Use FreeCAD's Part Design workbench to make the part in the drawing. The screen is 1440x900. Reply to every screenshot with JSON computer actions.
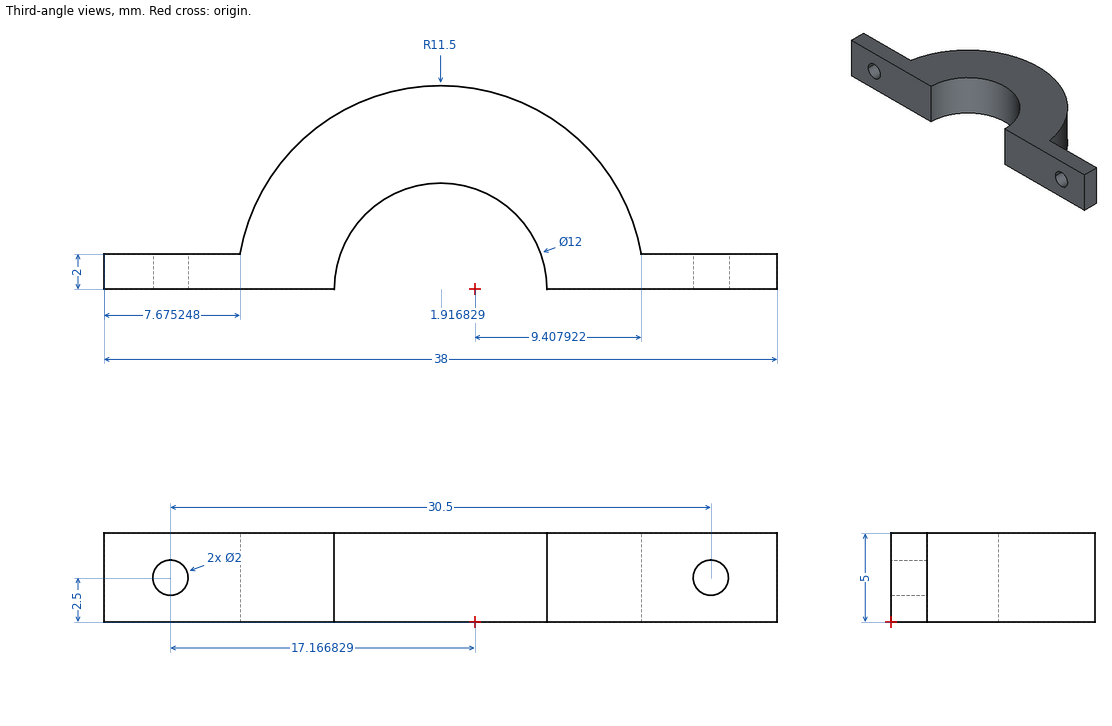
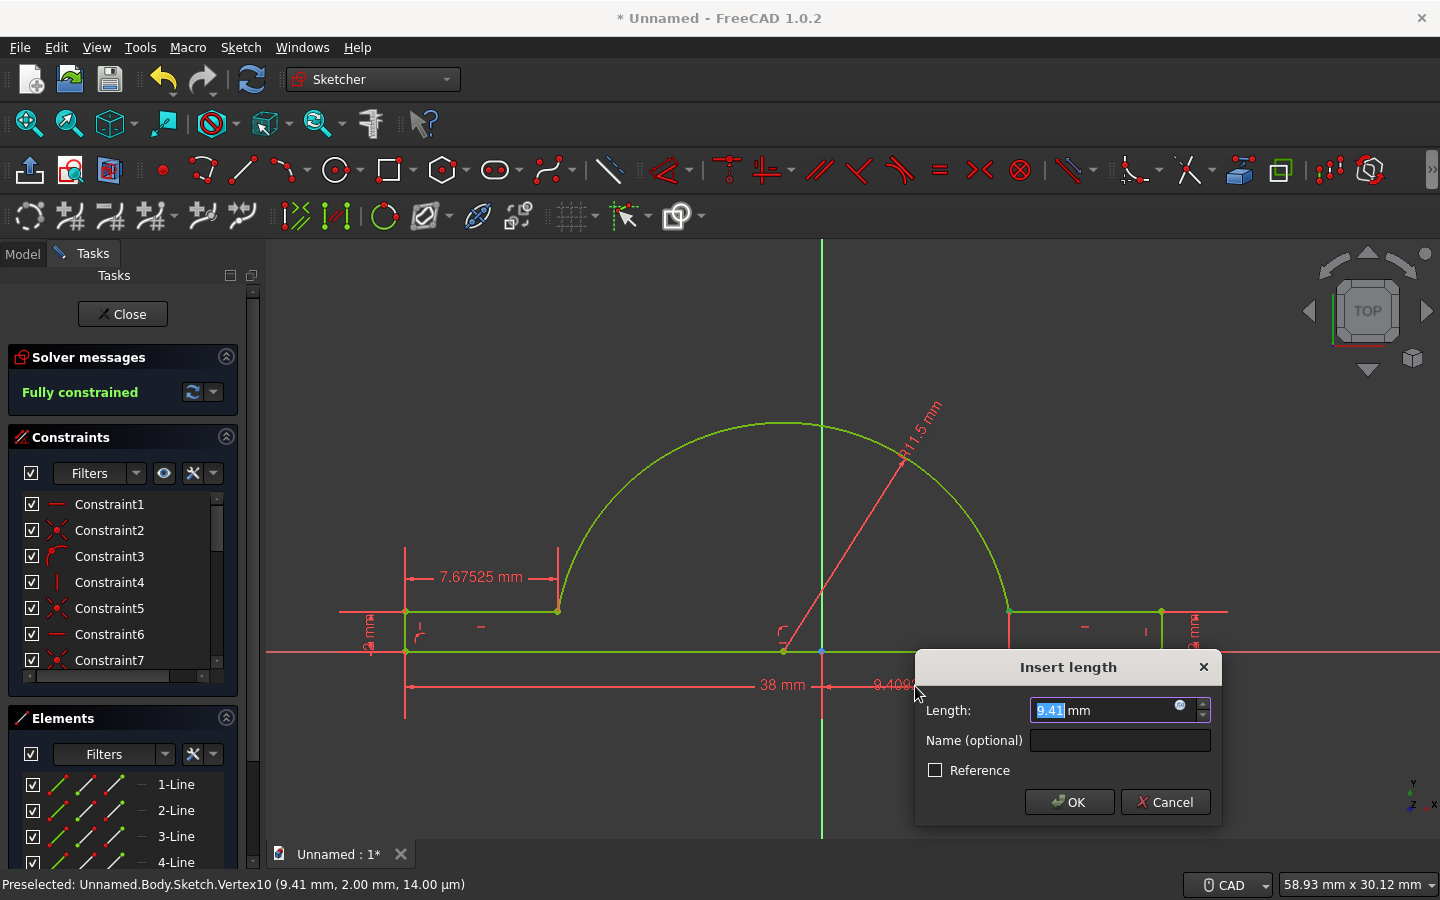
{"action": "type", "text": "9.407922"}
{"action": "key", "text": "Return"}
{"action": "key", "text": "Escape"}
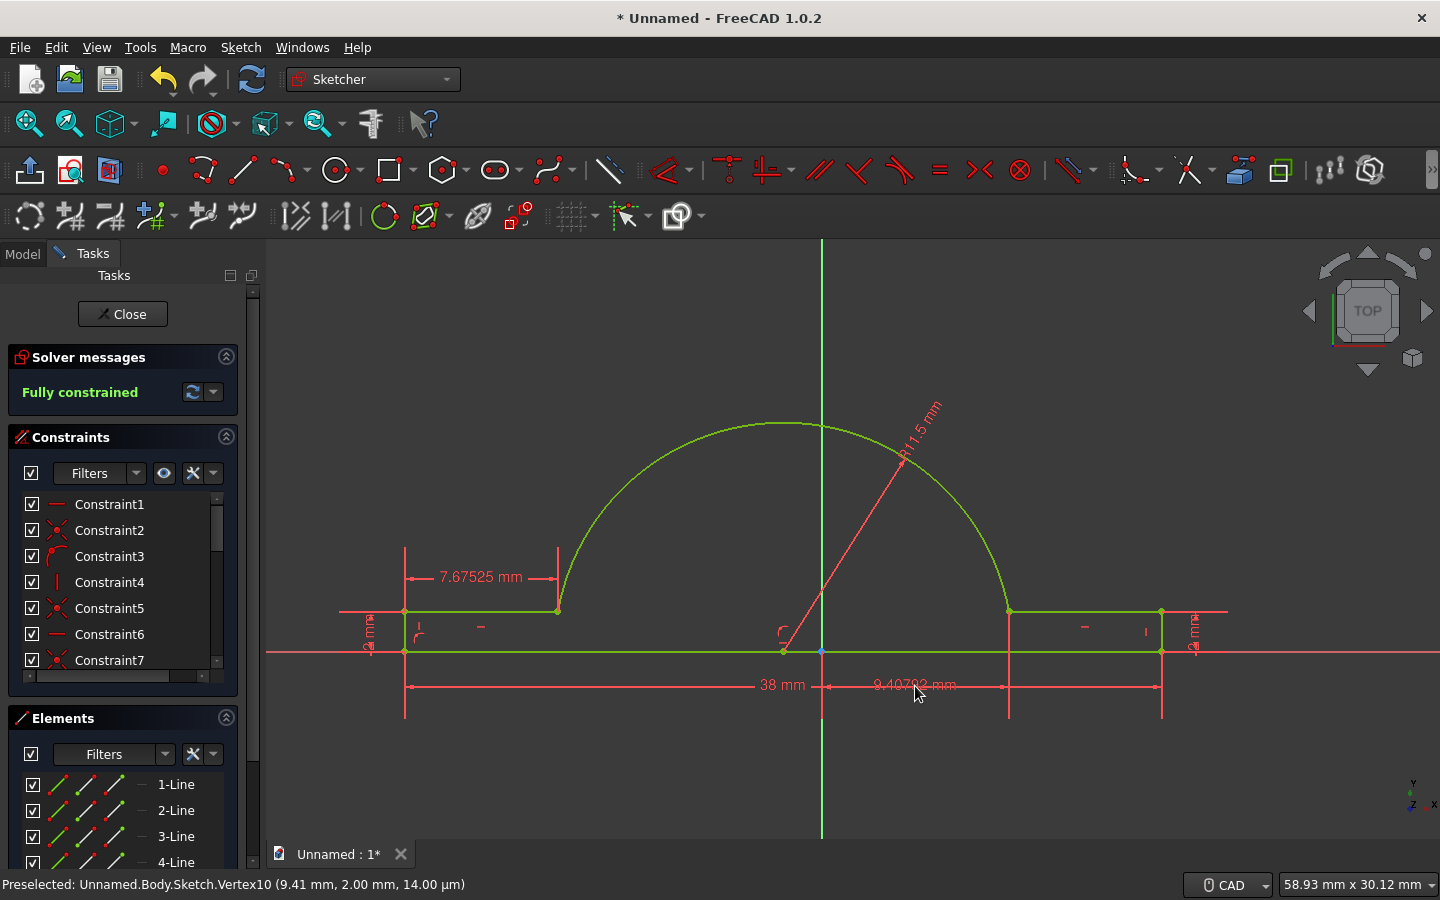
{"action": "left_click", "coordinate": [123, 314]}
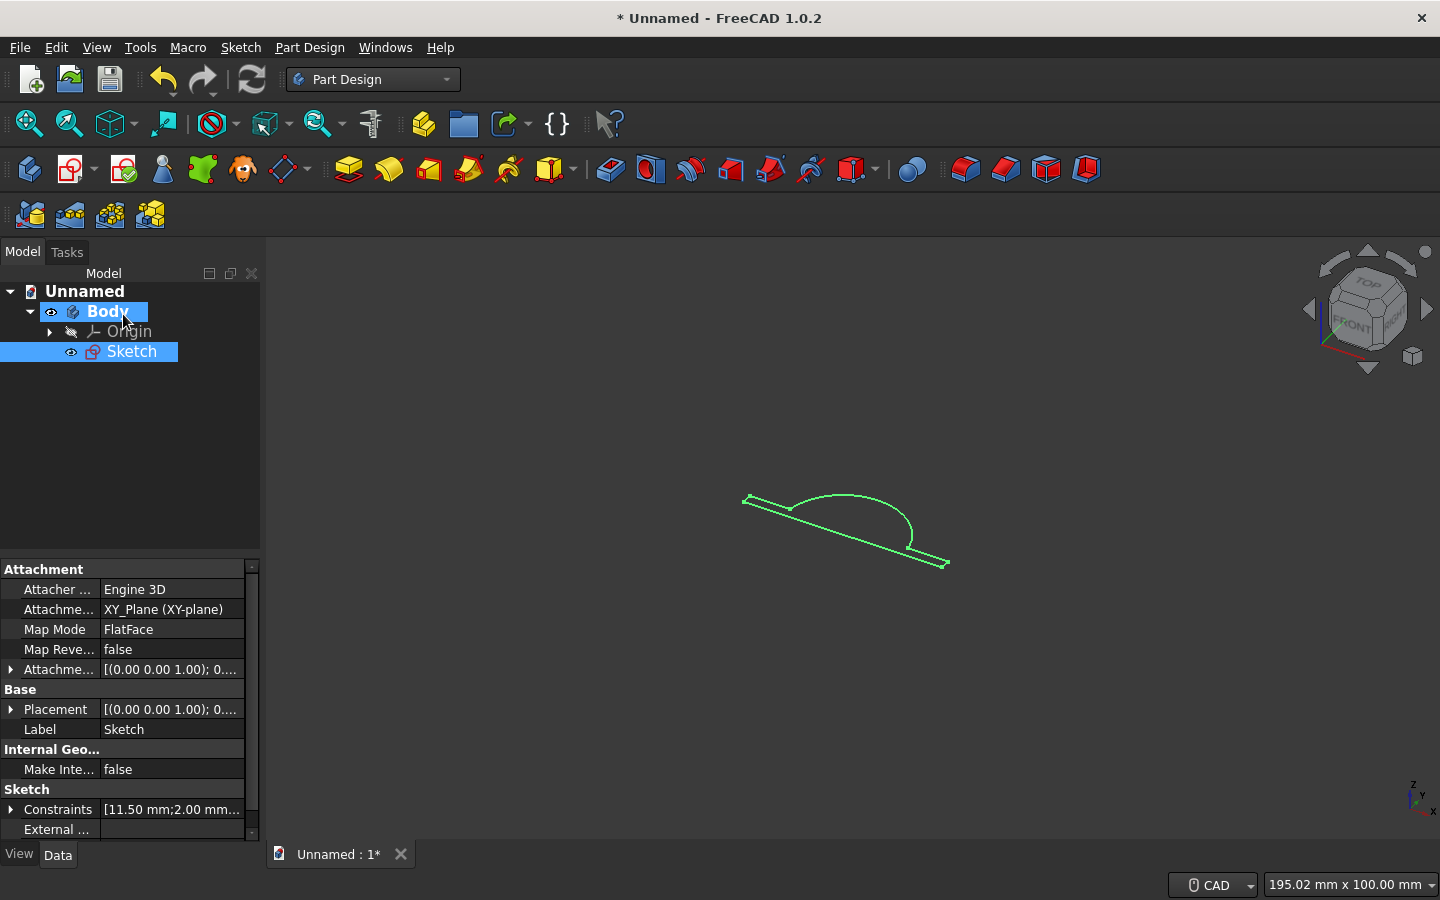
{"action": "left_click", "coordinate": [350, 170]}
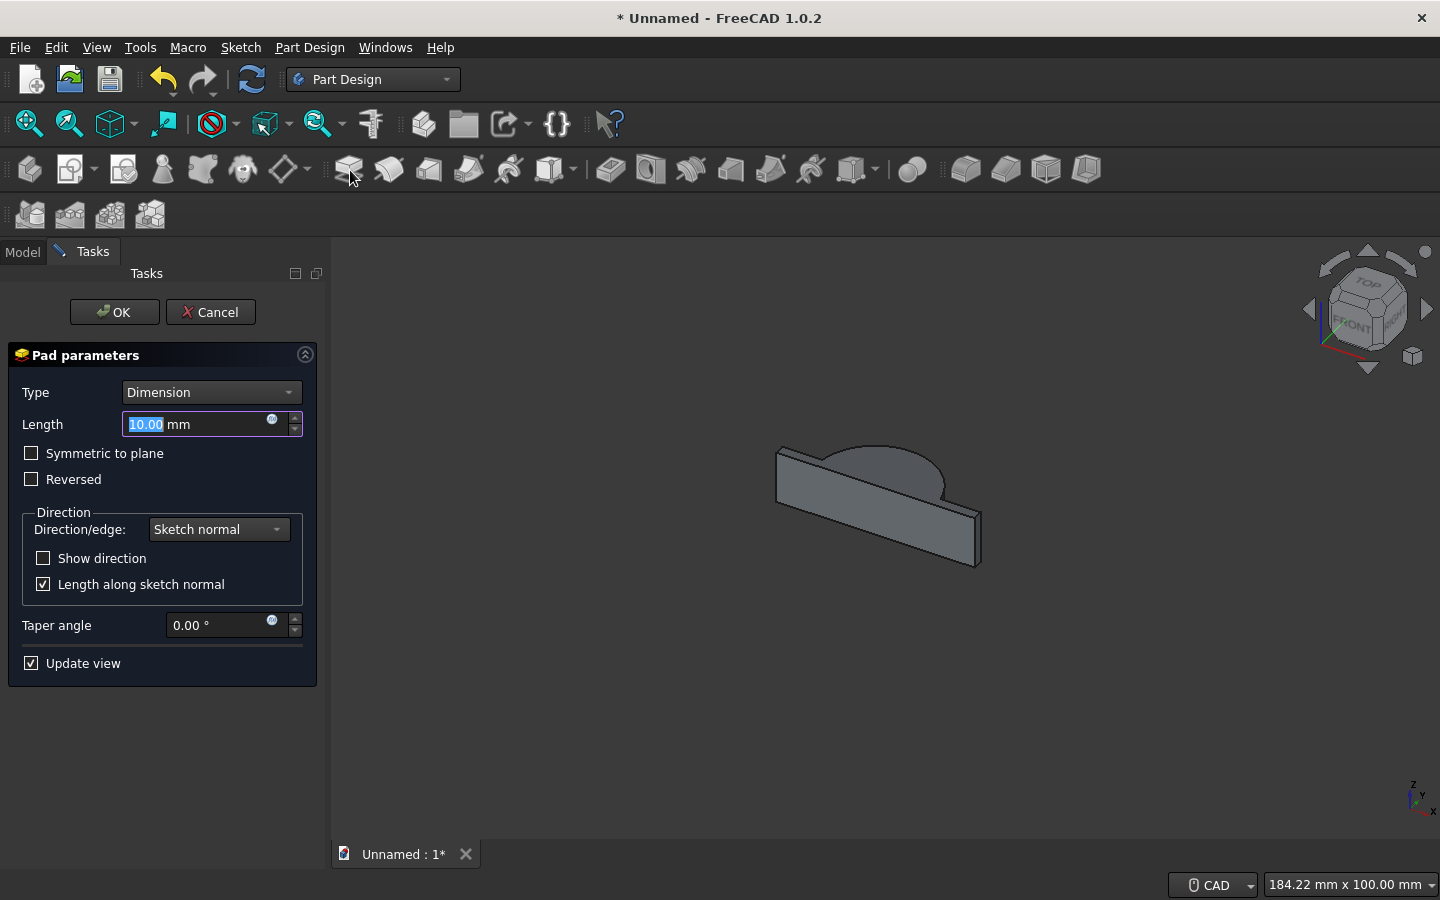
{"action": "type", "text": "5"}
{"action": "key", "text": "Tab"}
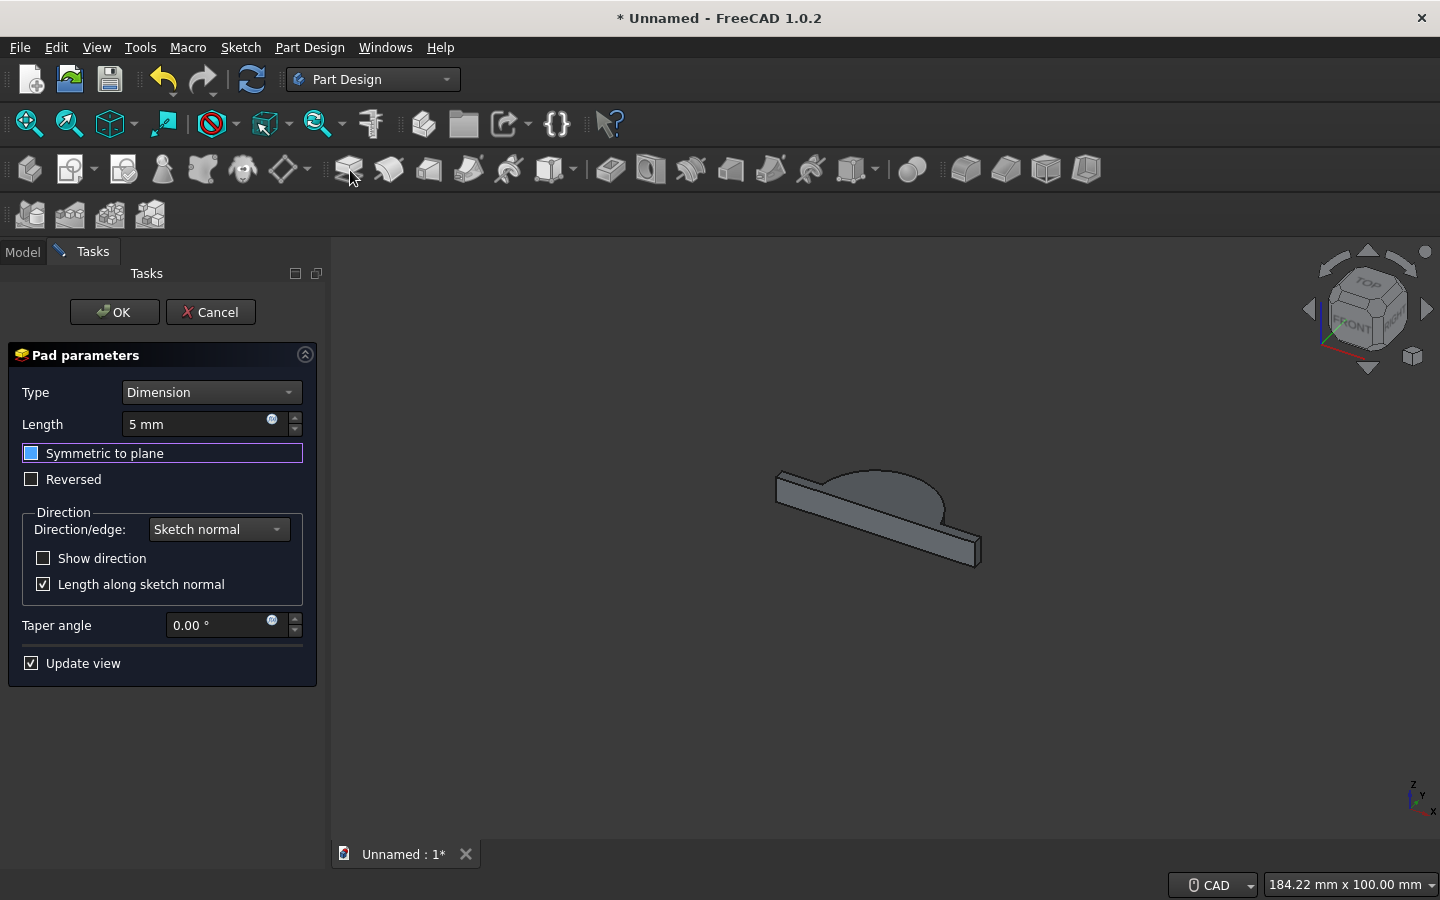
{"action": "left_click", "coordinate": [115, 312]}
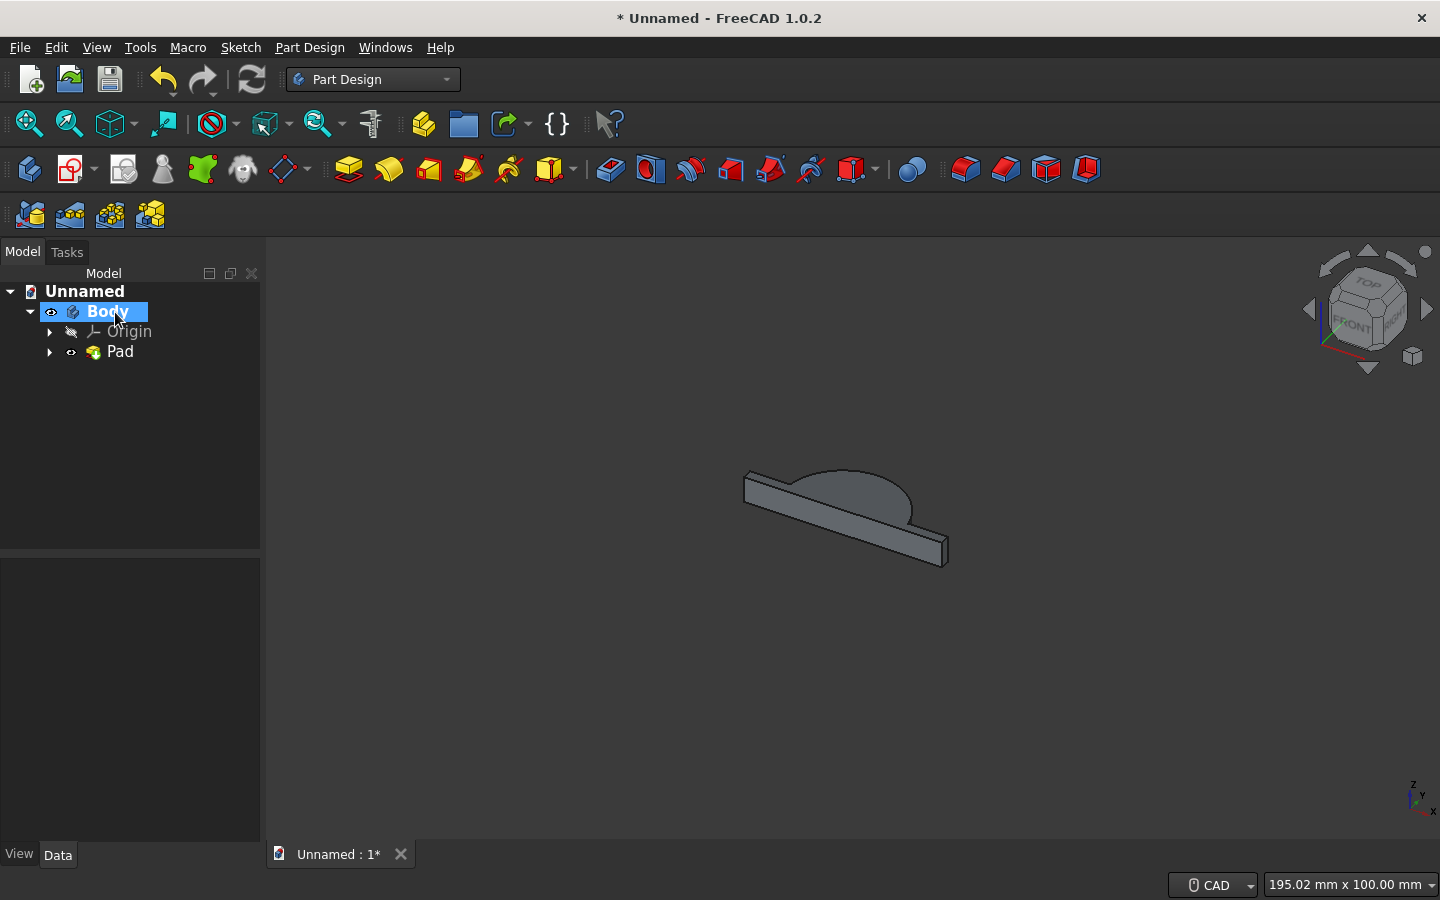
{"action": "left_click", "coordinate": [30, 124]}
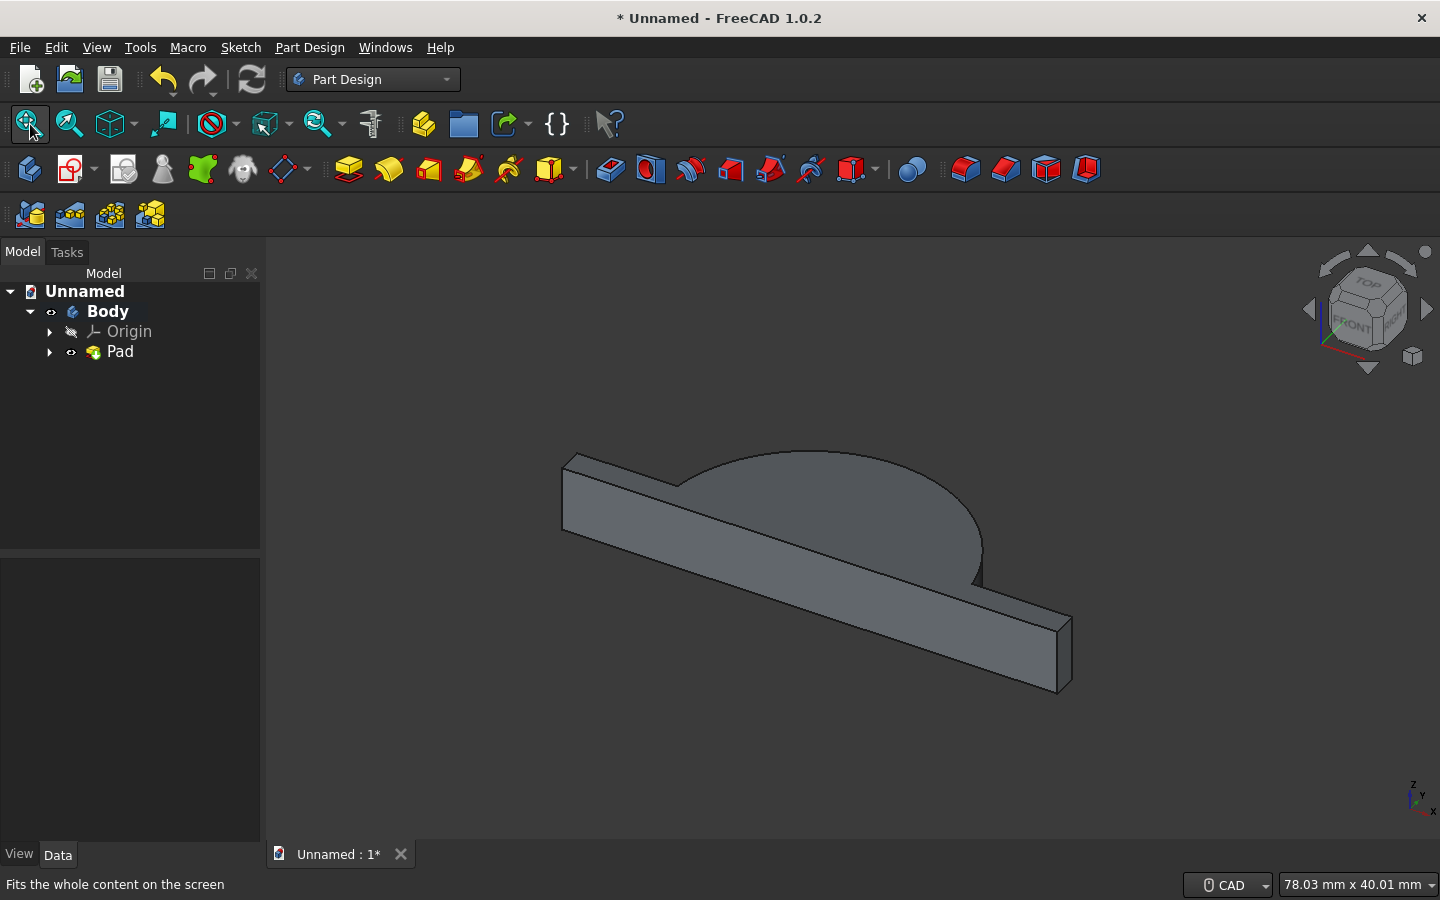
{"action": "key", "text": "4"}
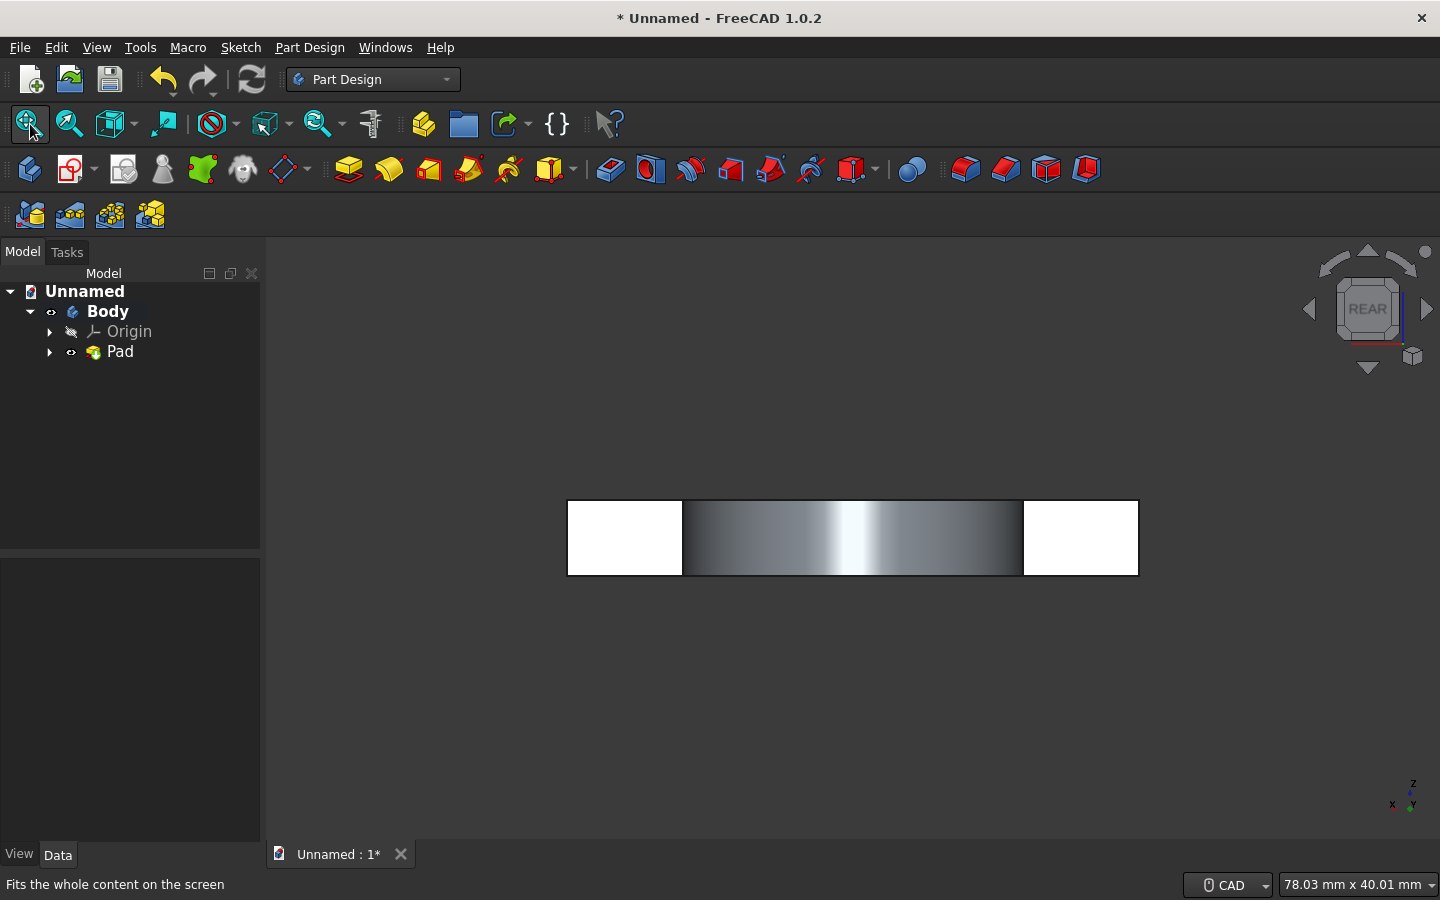
{"action": "left_click", "coordinate": [608, 537]}